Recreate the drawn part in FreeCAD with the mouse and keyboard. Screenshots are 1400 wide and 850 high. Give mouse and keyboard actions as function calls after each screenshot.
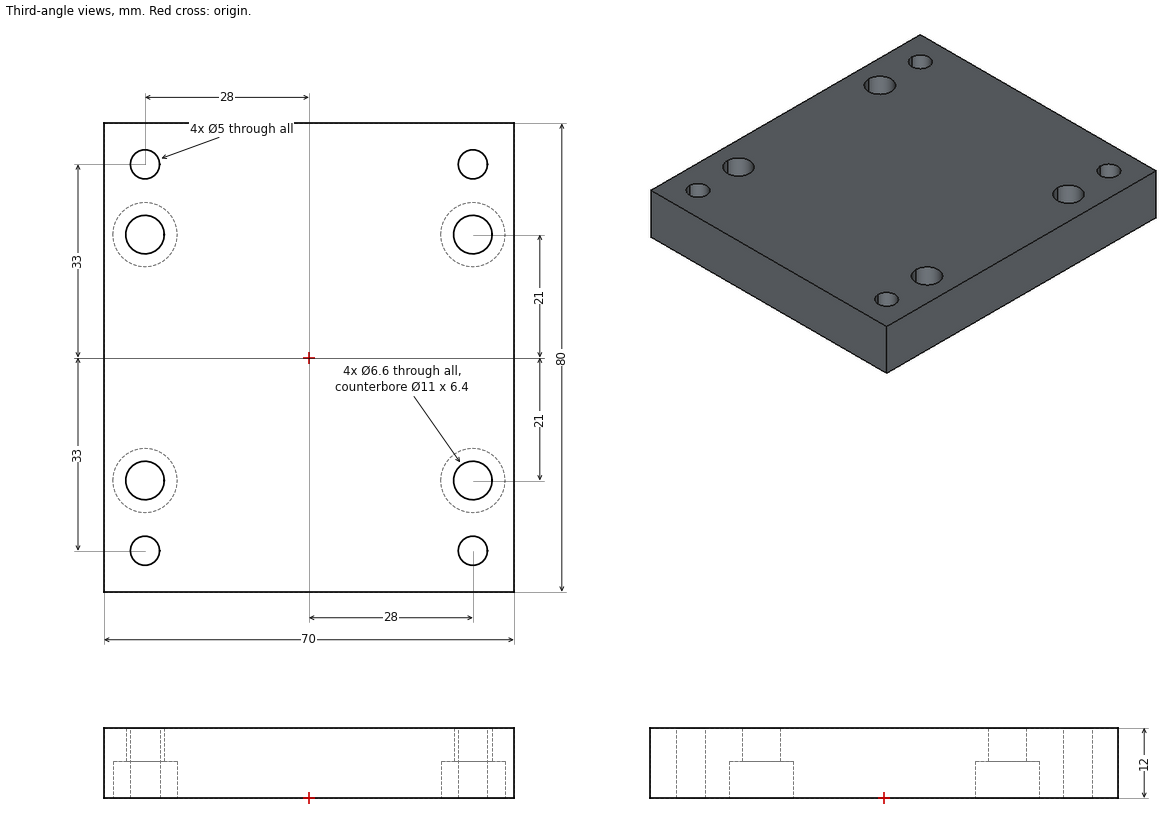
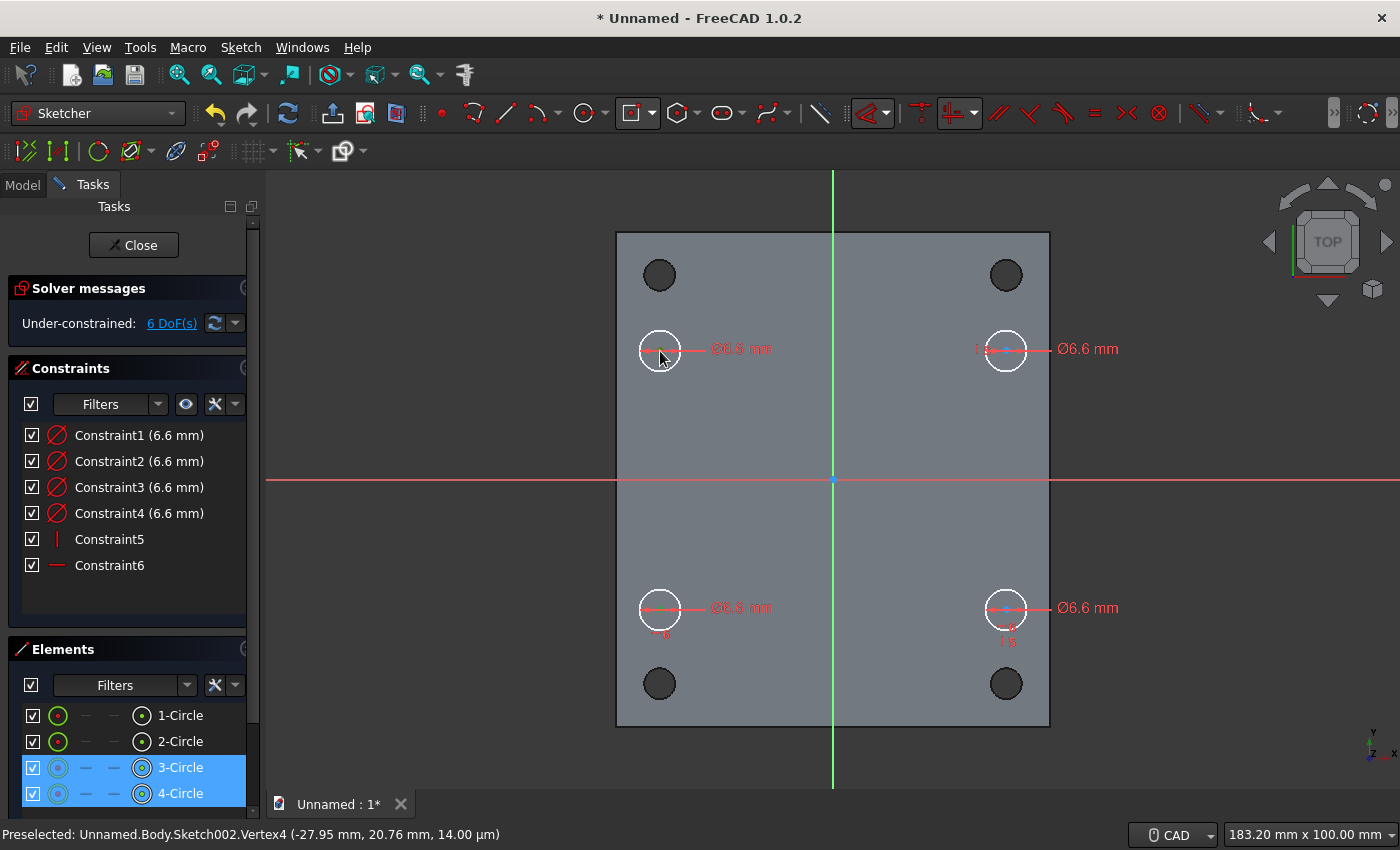
click(976, 114)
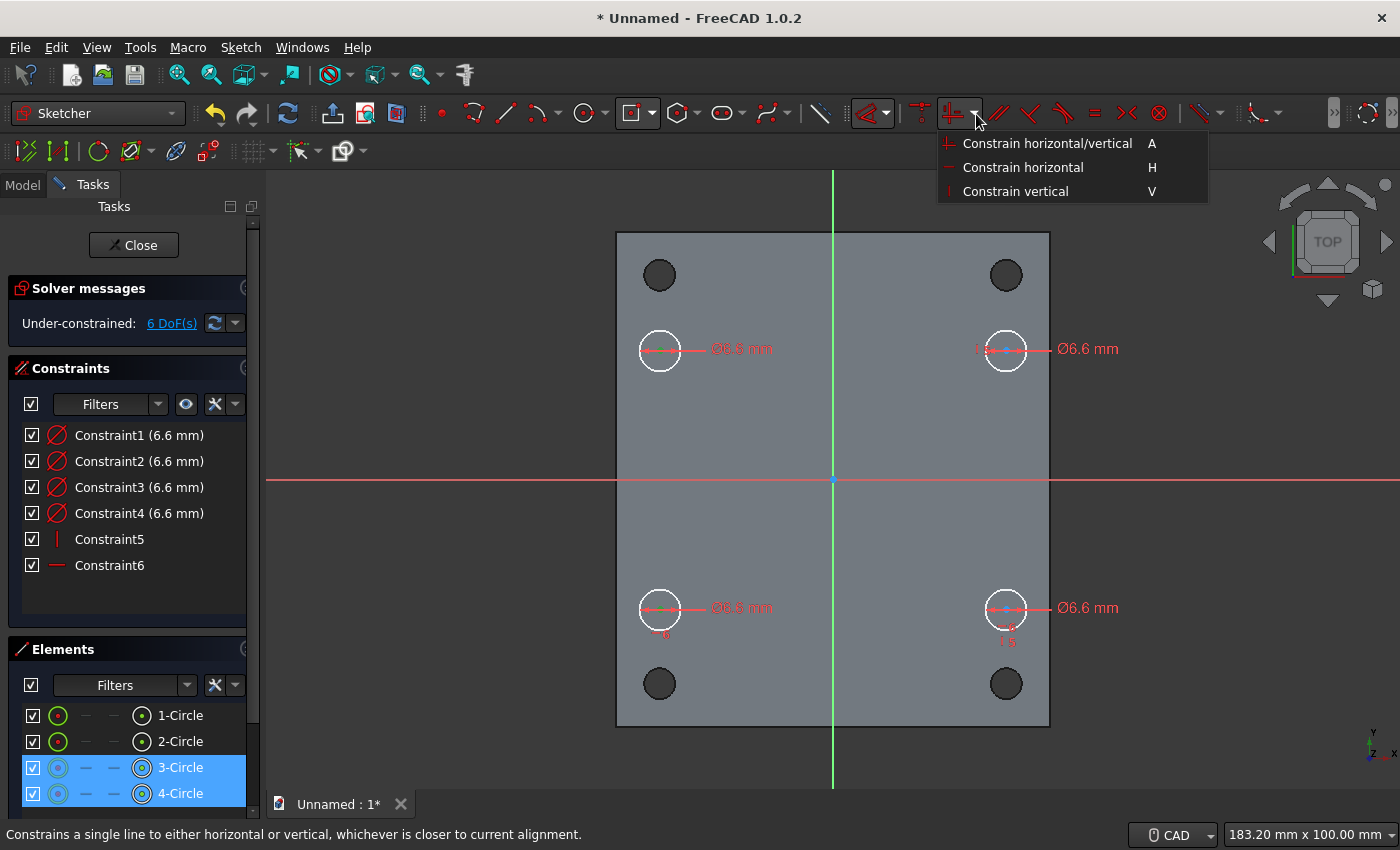
click(1073, 191)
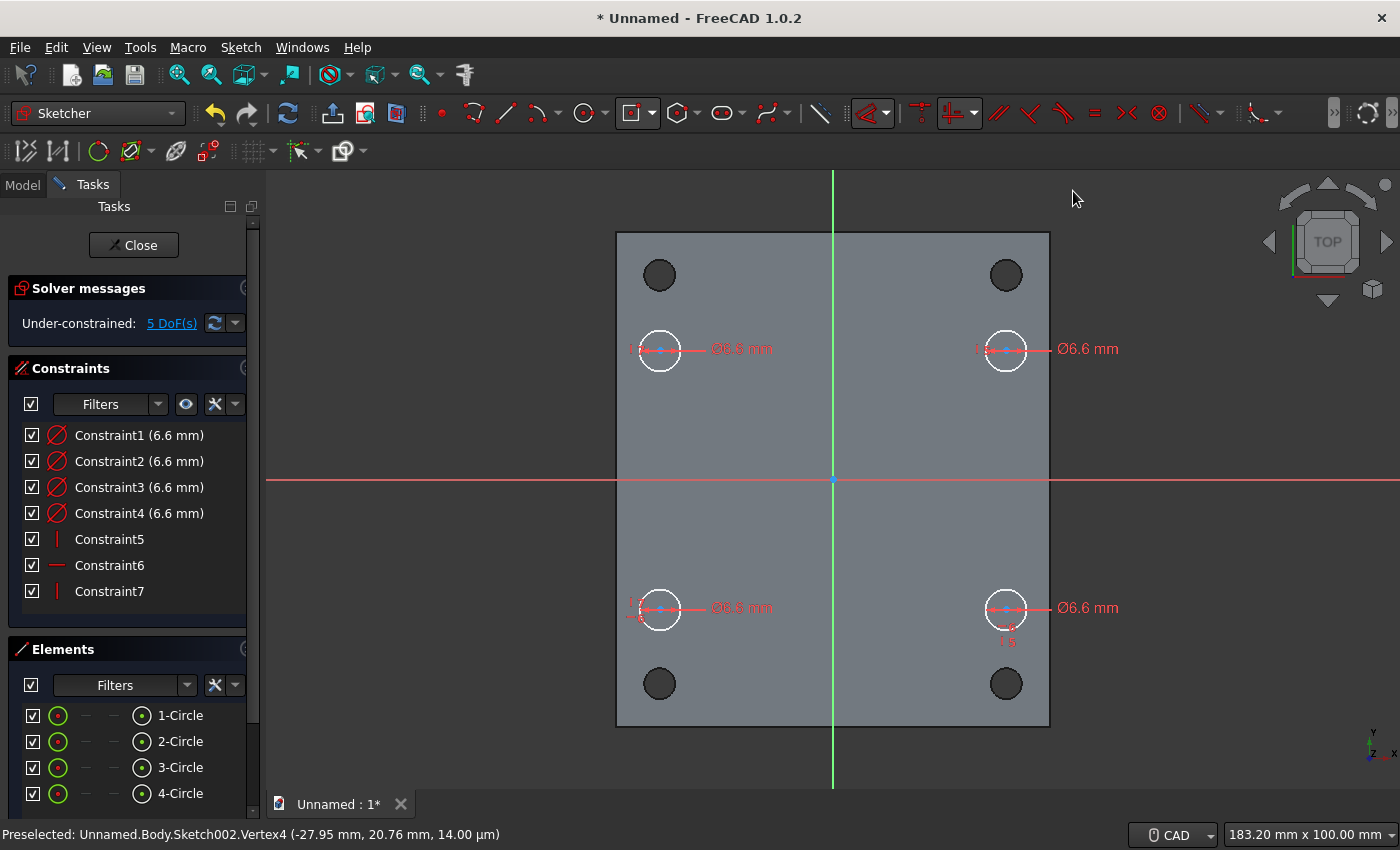
click(1006, 351)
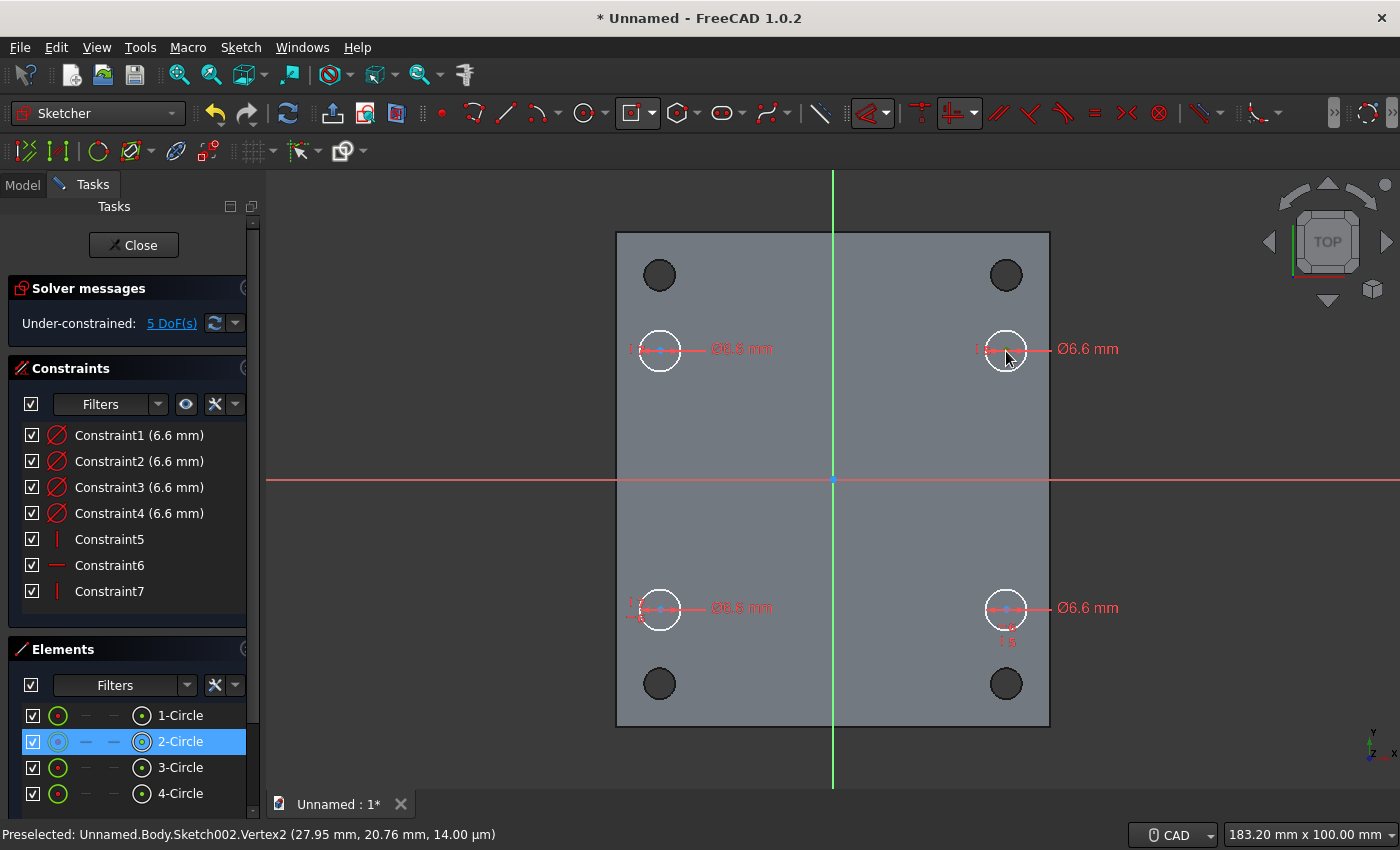
click(660, 351)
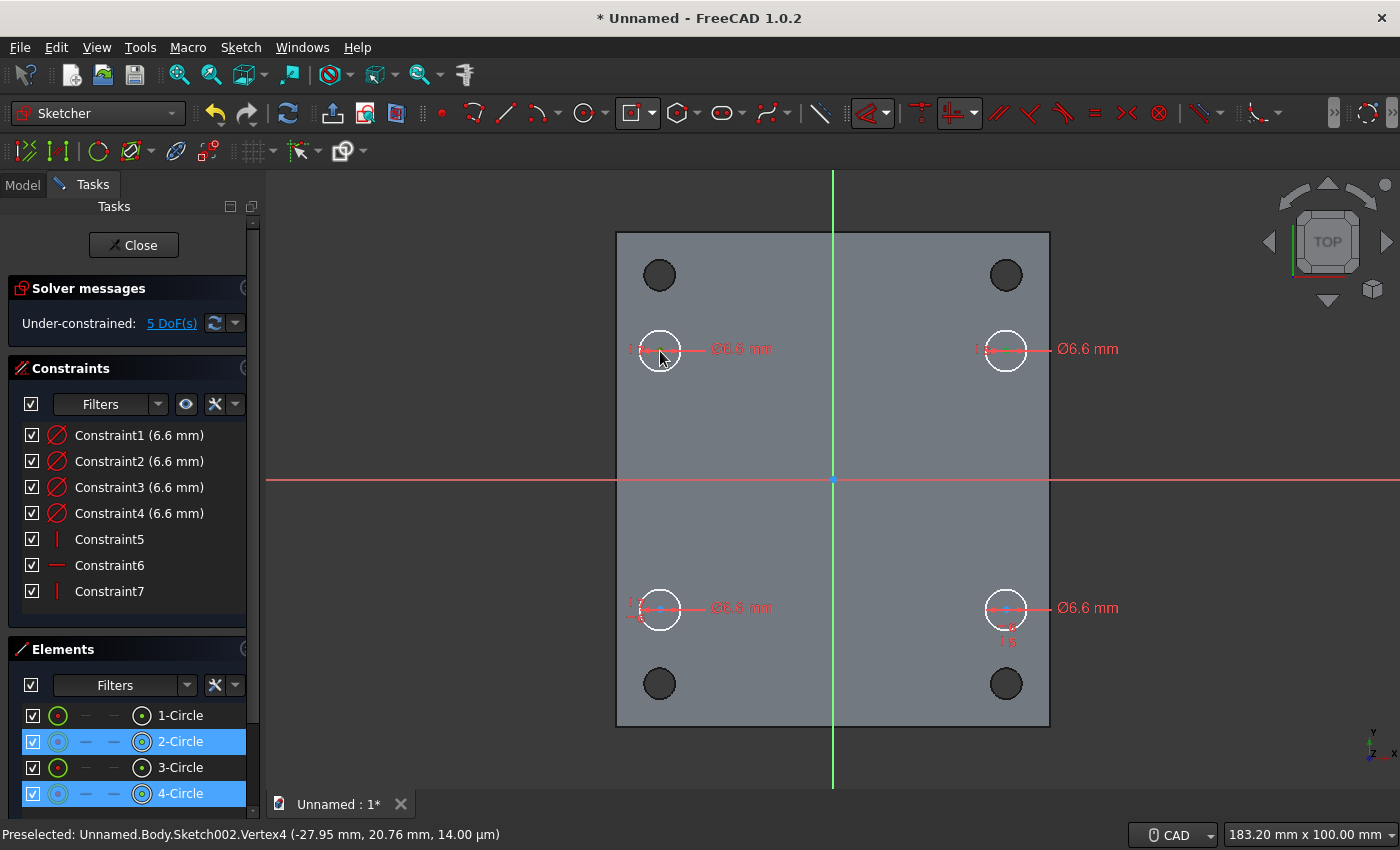
click(976, 114)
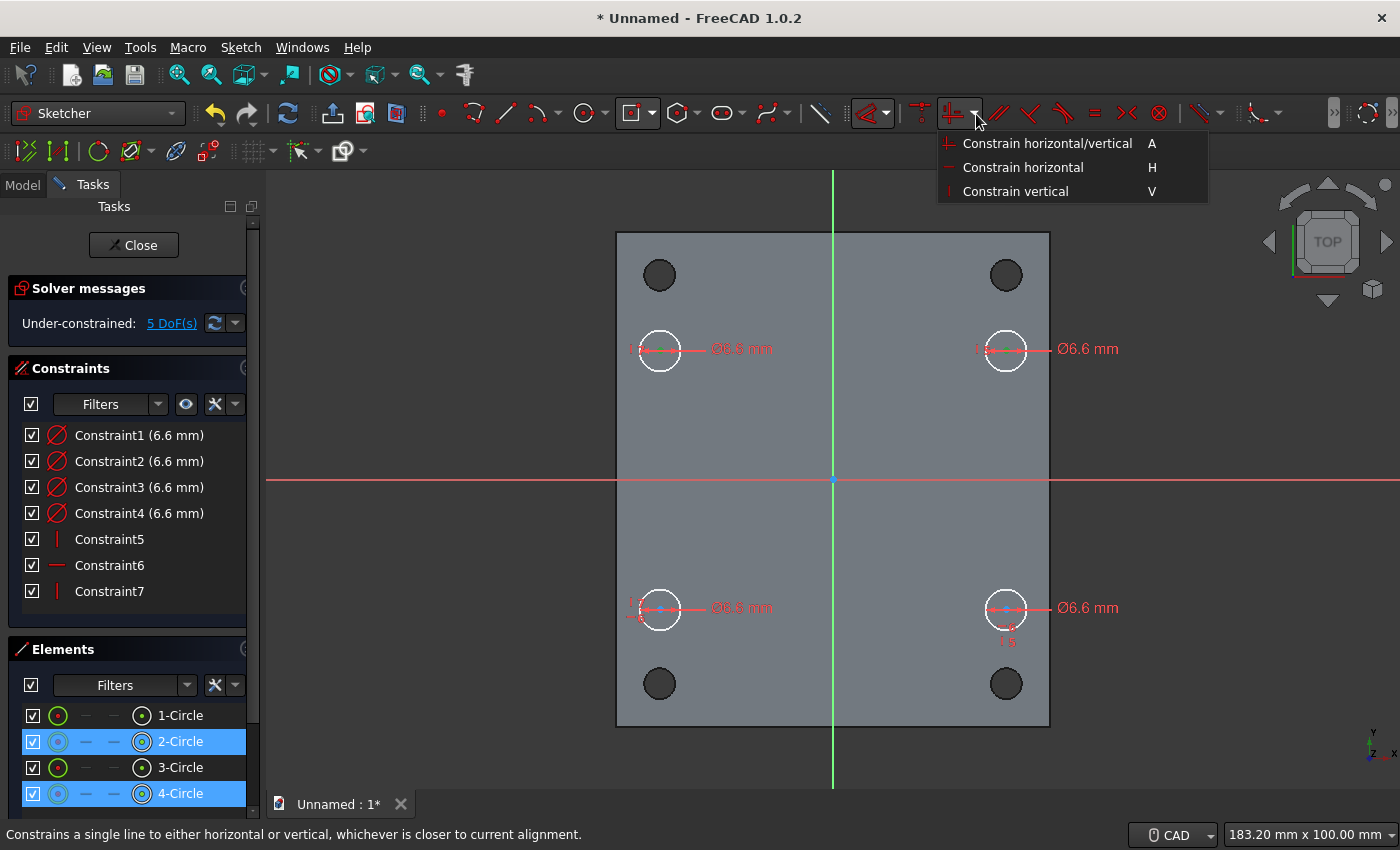
click(1073, 167)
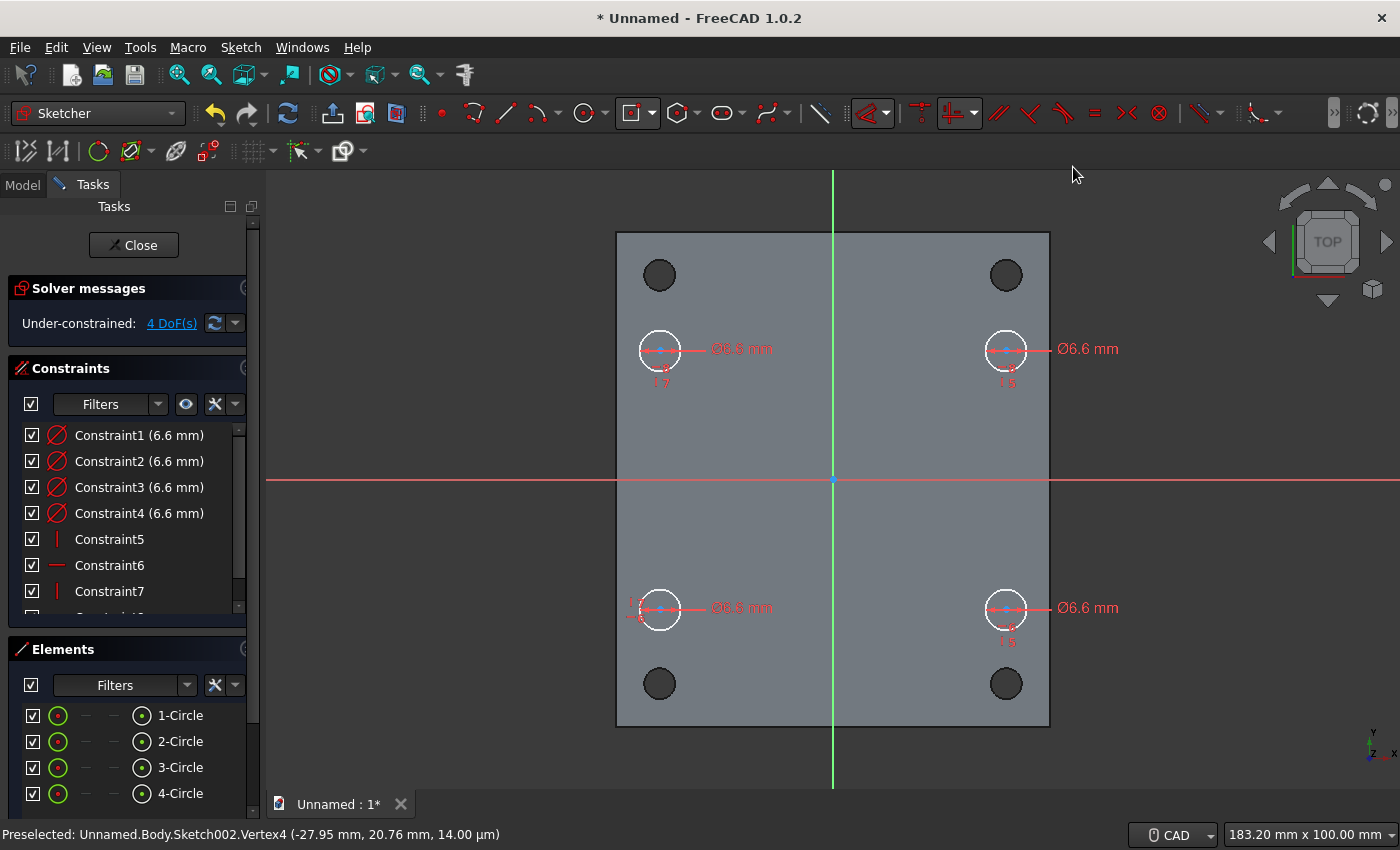
click(1006, 610)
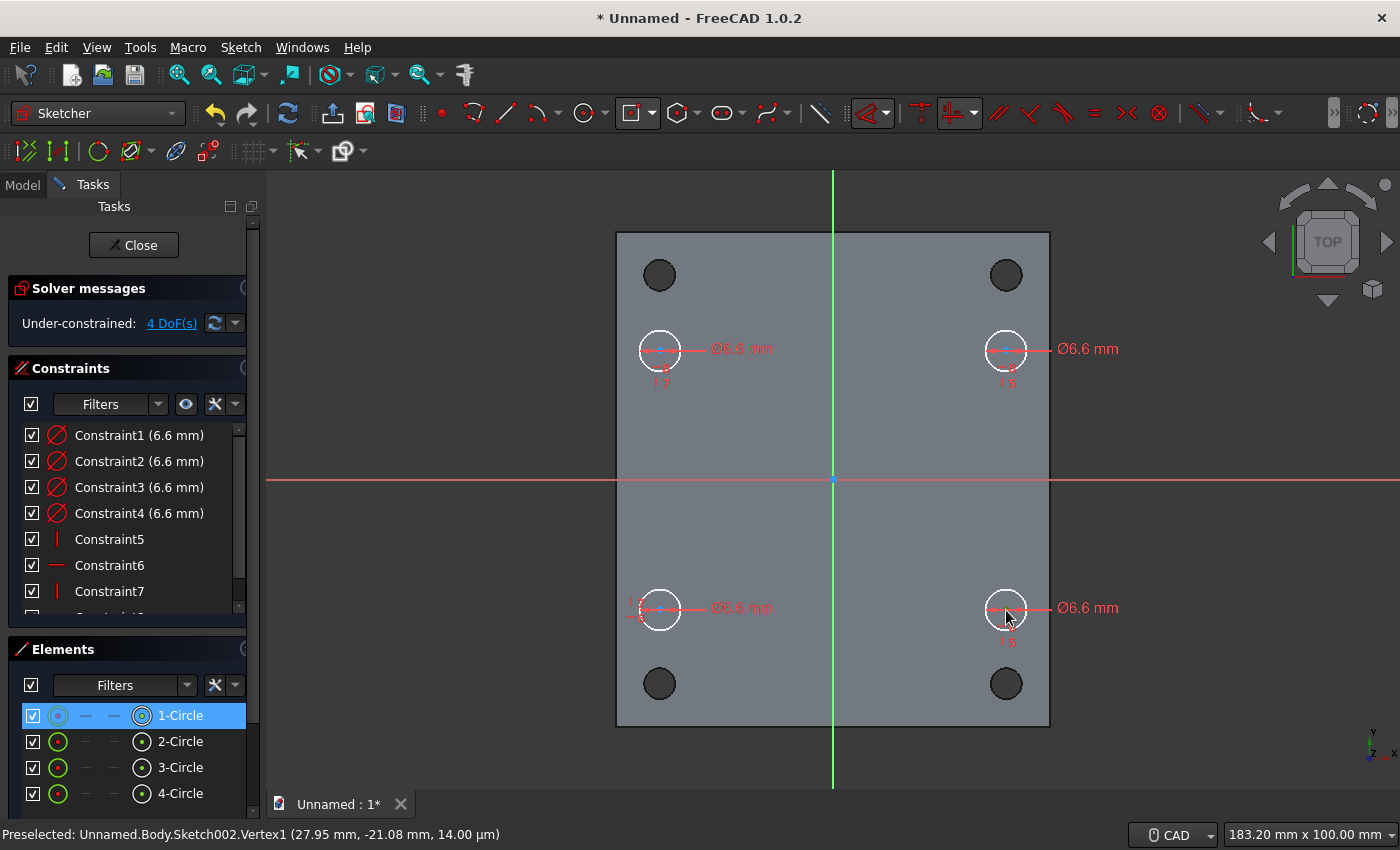
key(l)